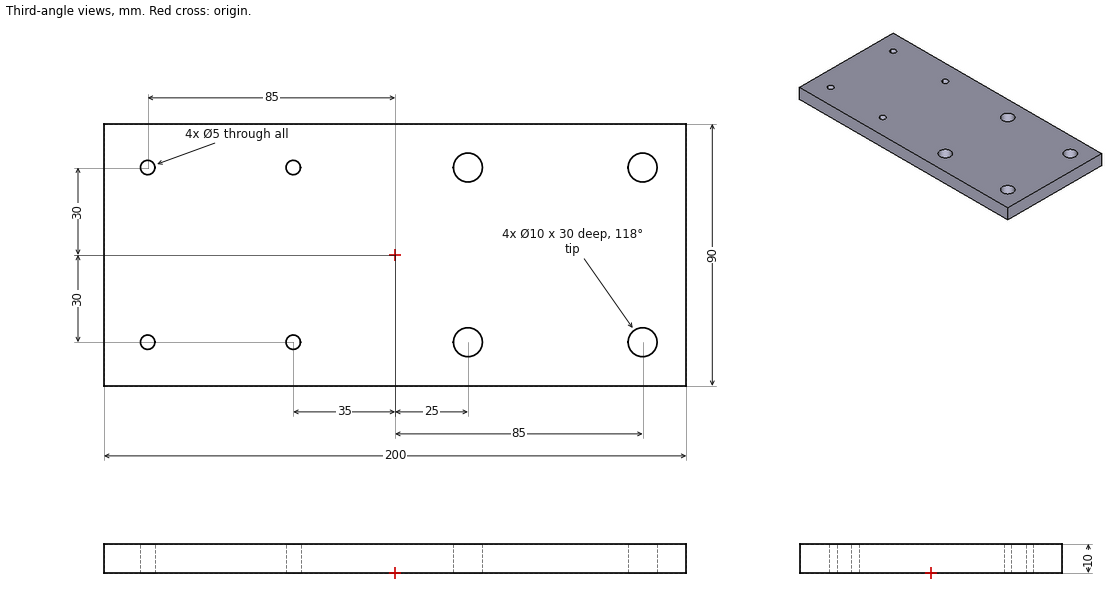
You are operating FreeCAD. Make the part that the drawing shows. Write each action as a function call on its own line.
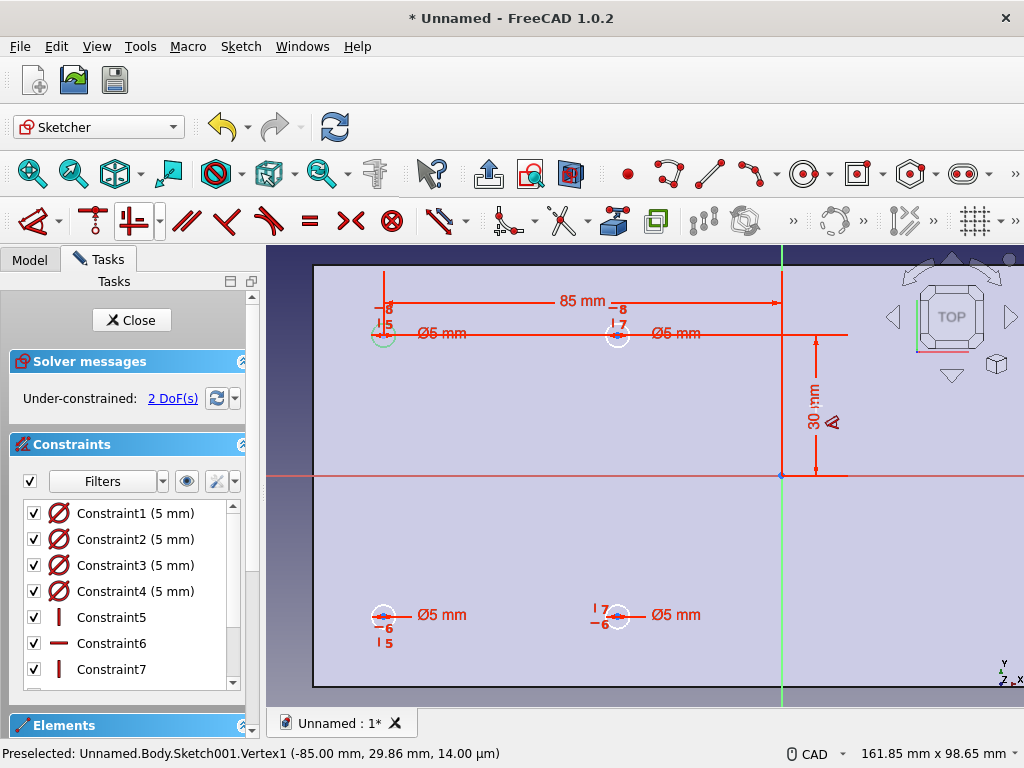
click(618, 617)
click(700, 651)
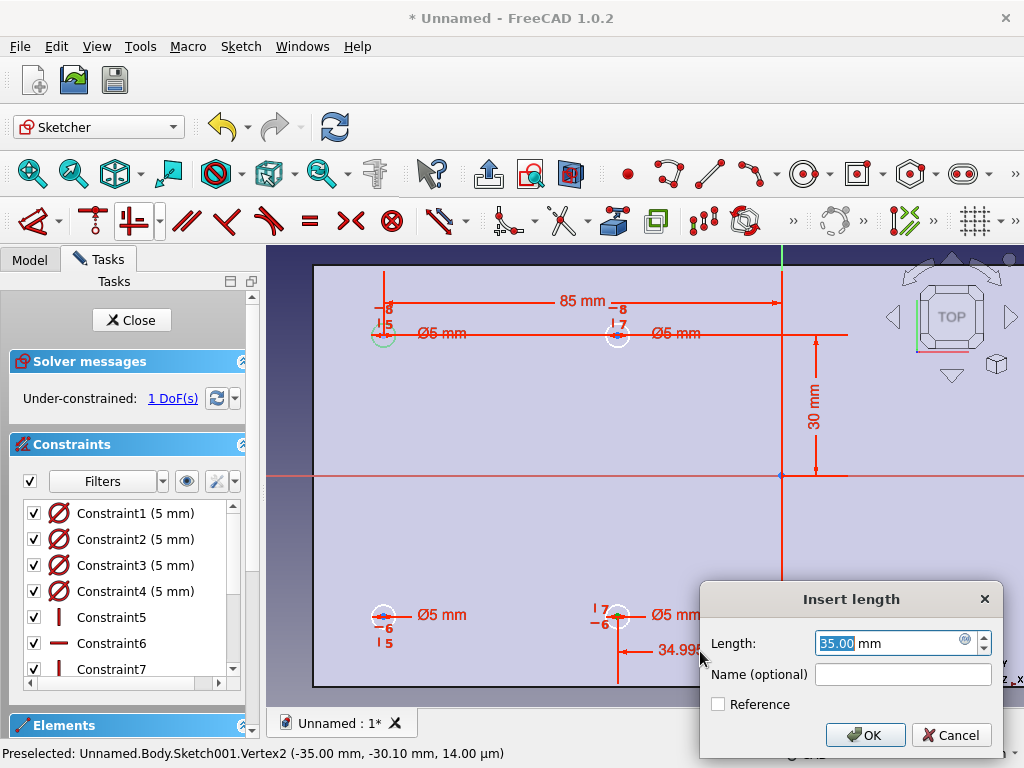
text(35)
key(Return)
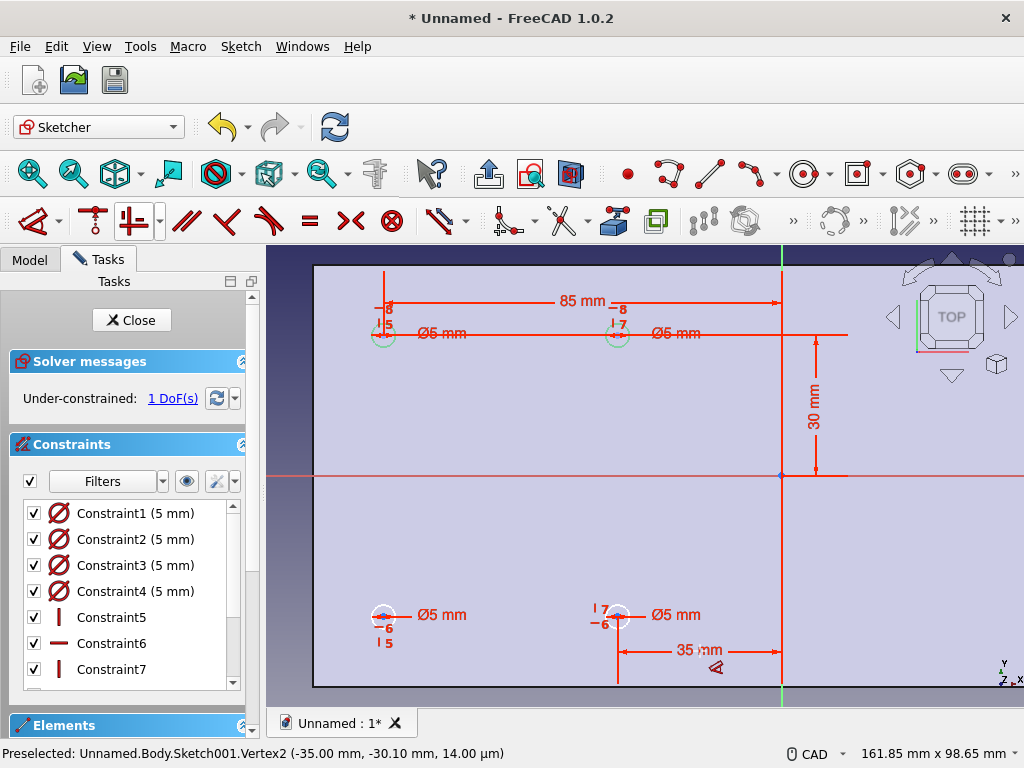
click(618, 617)
click(816, 546)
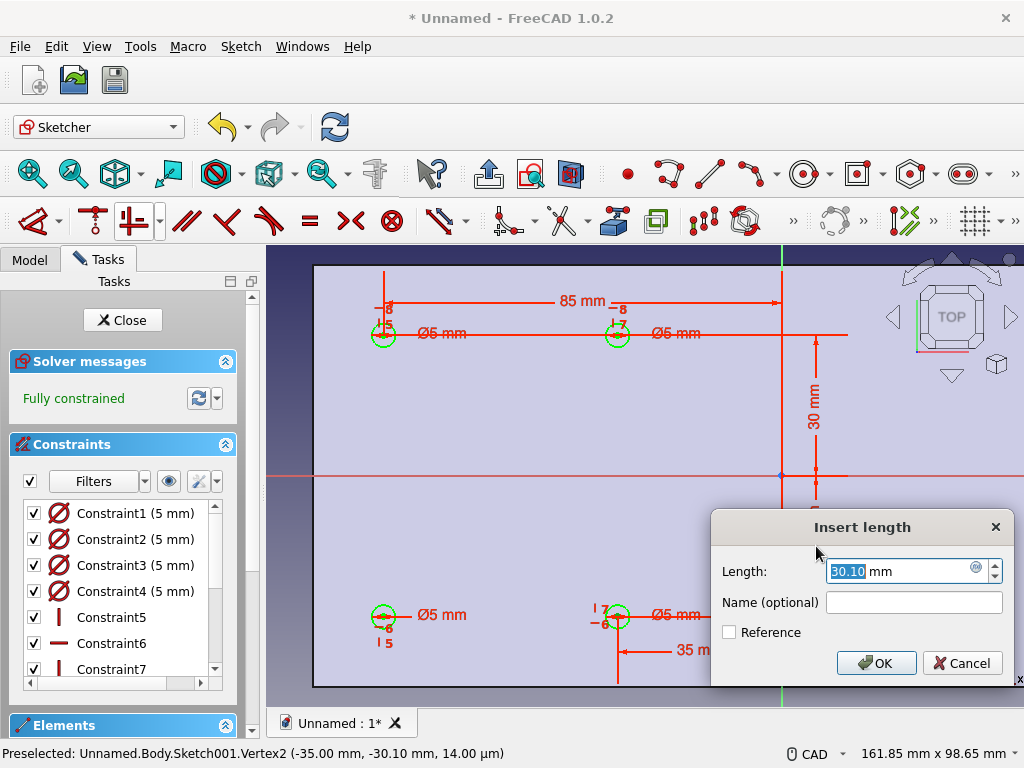
text(30)
key(Return)
key(Escape)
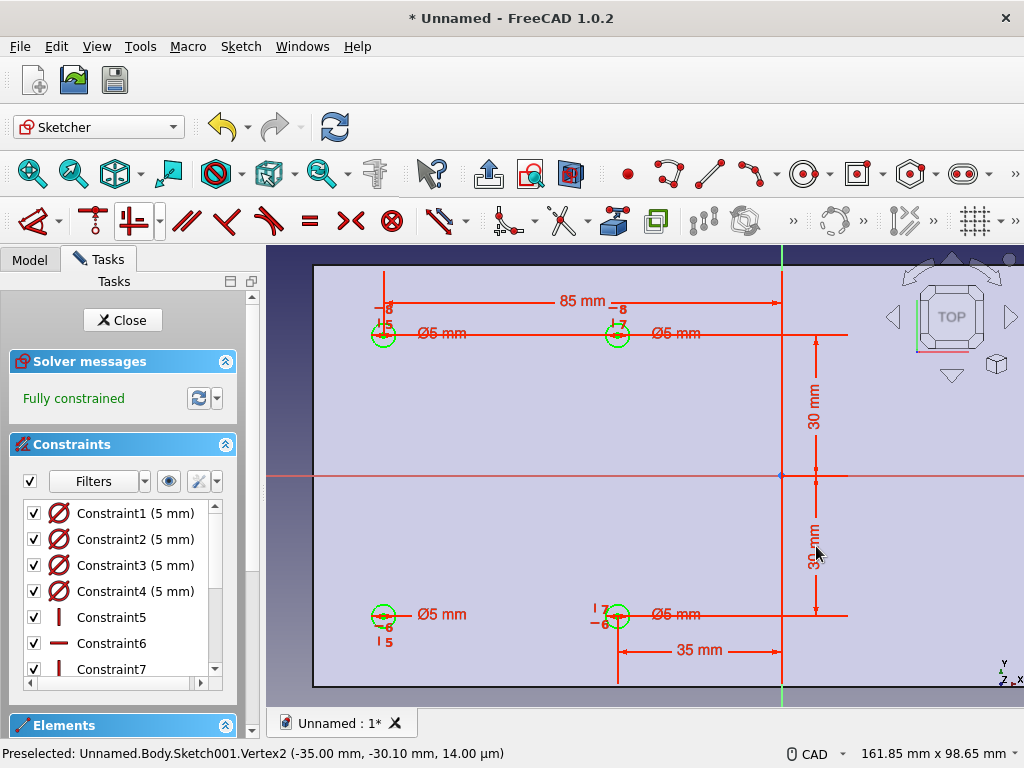
click(123, 320)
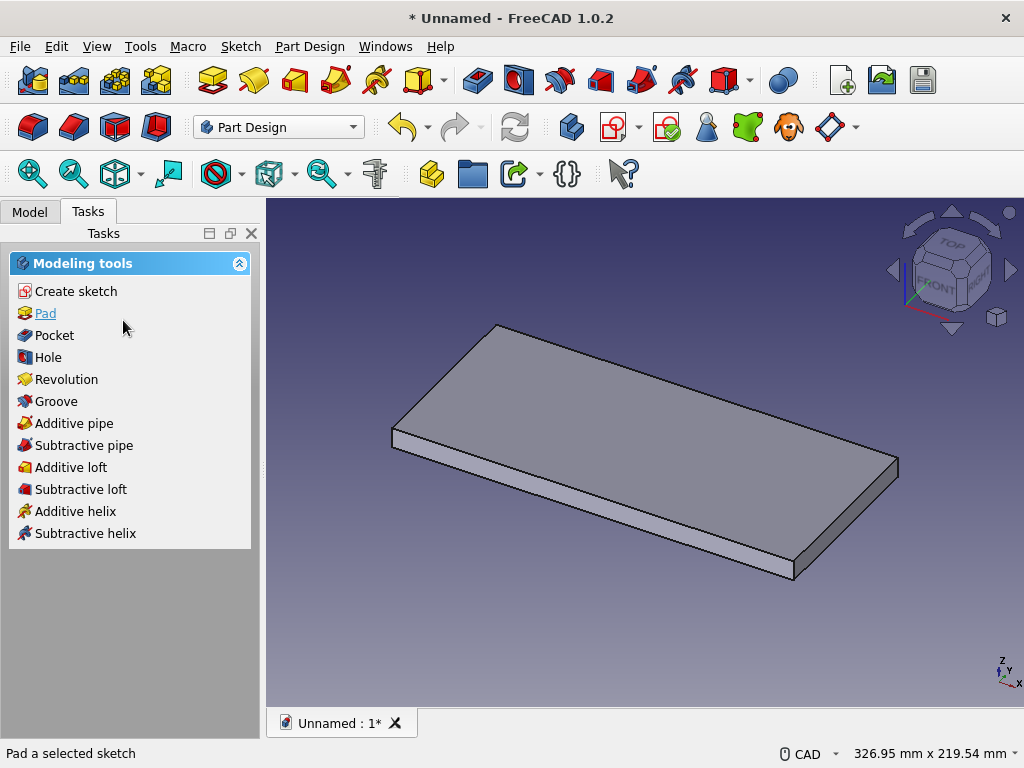
click(519, 80)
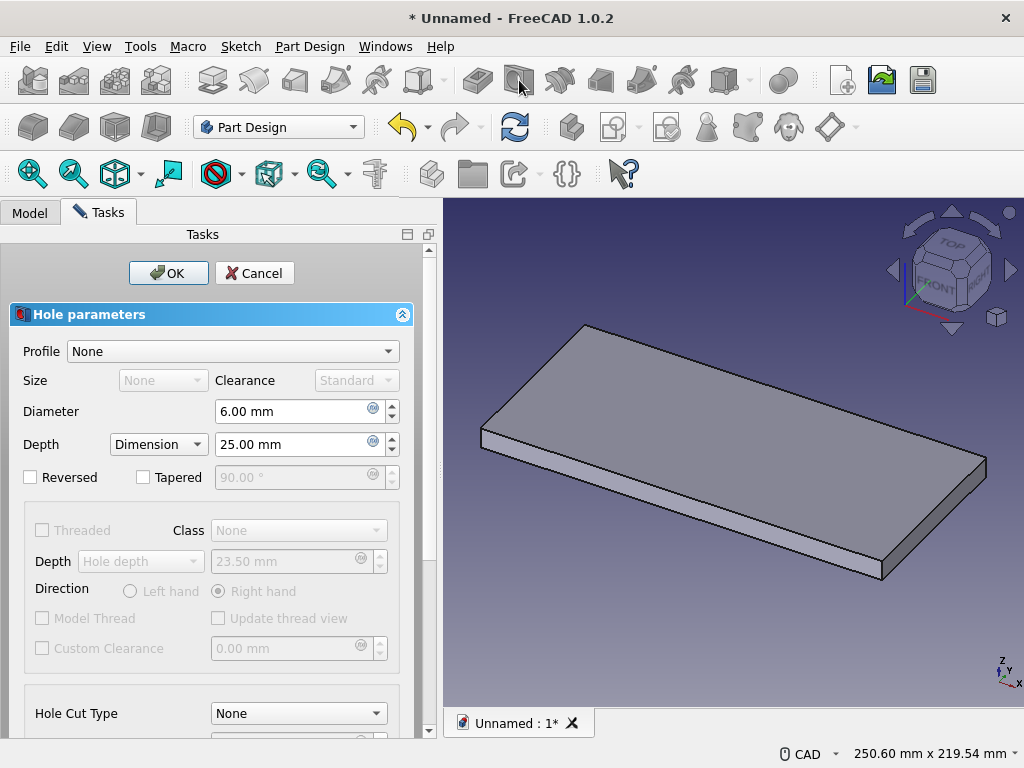
triple_click(300, 412)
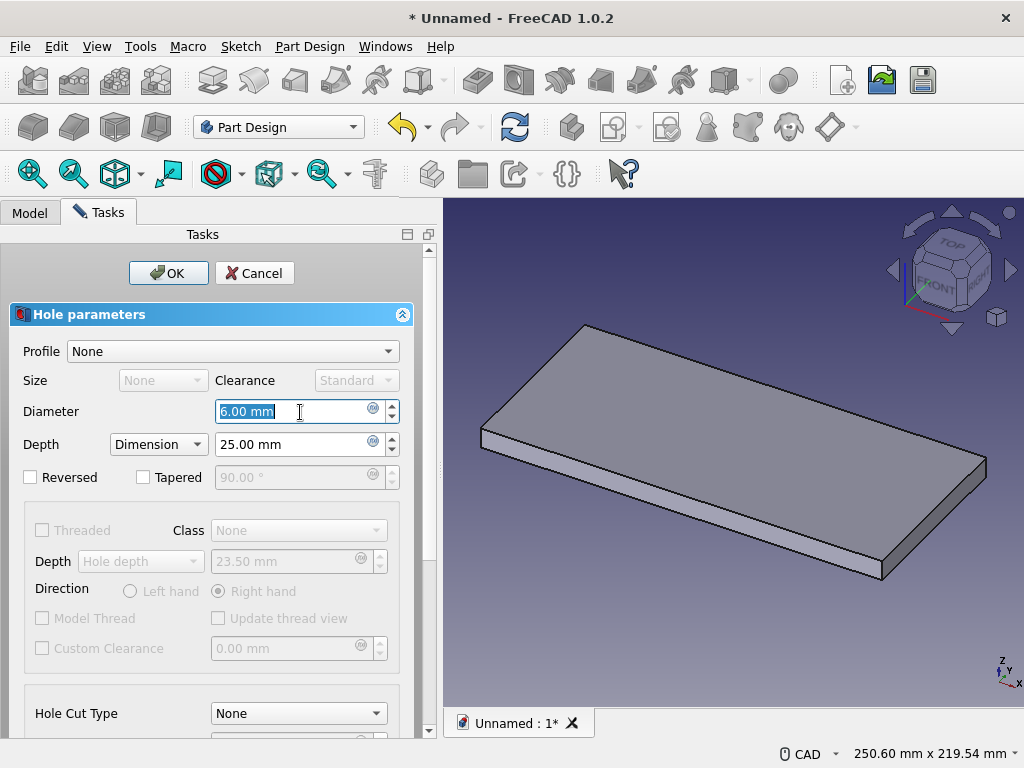
text(5)
key(Tab)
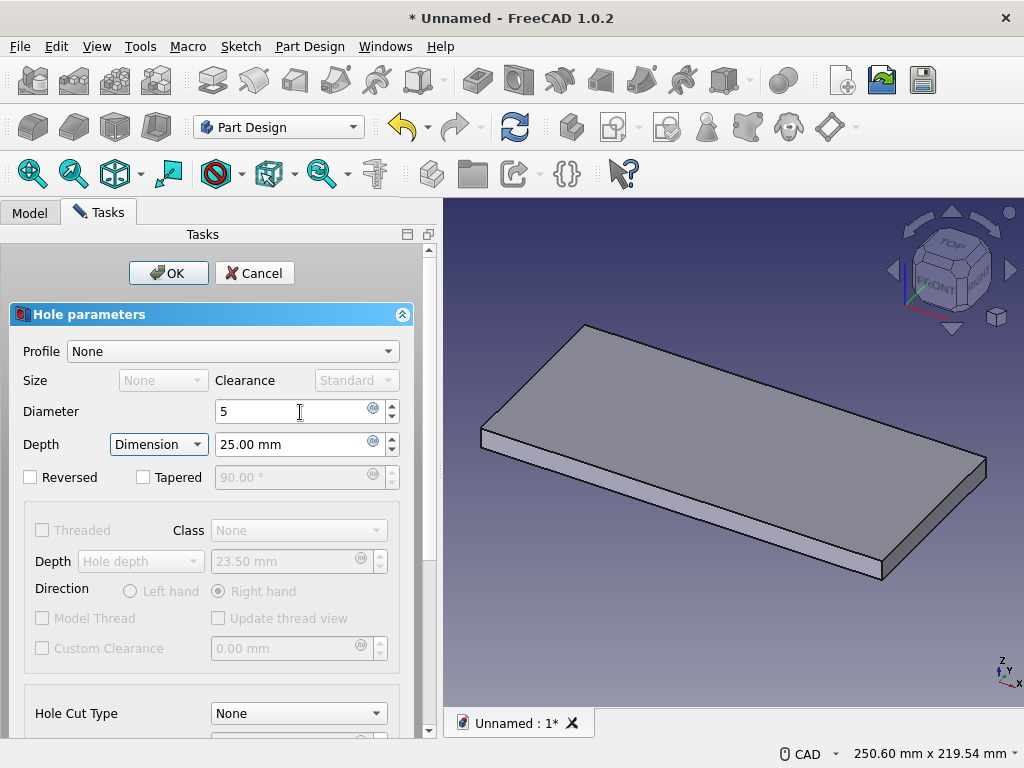
click(160, 444)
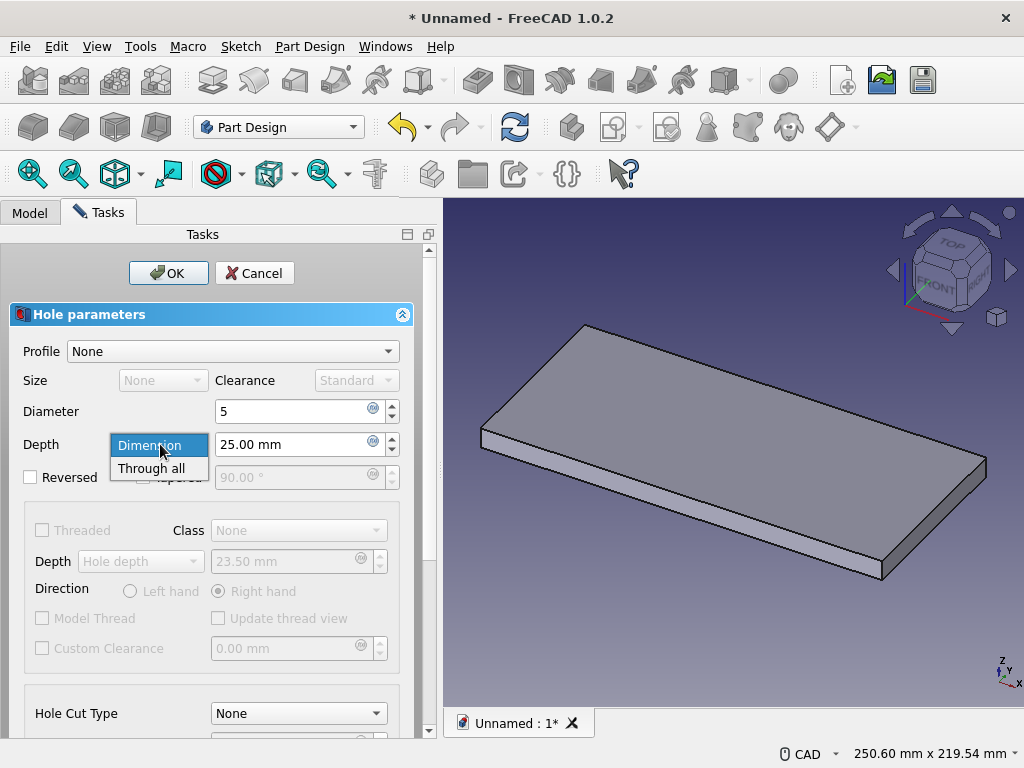
click(158, 468)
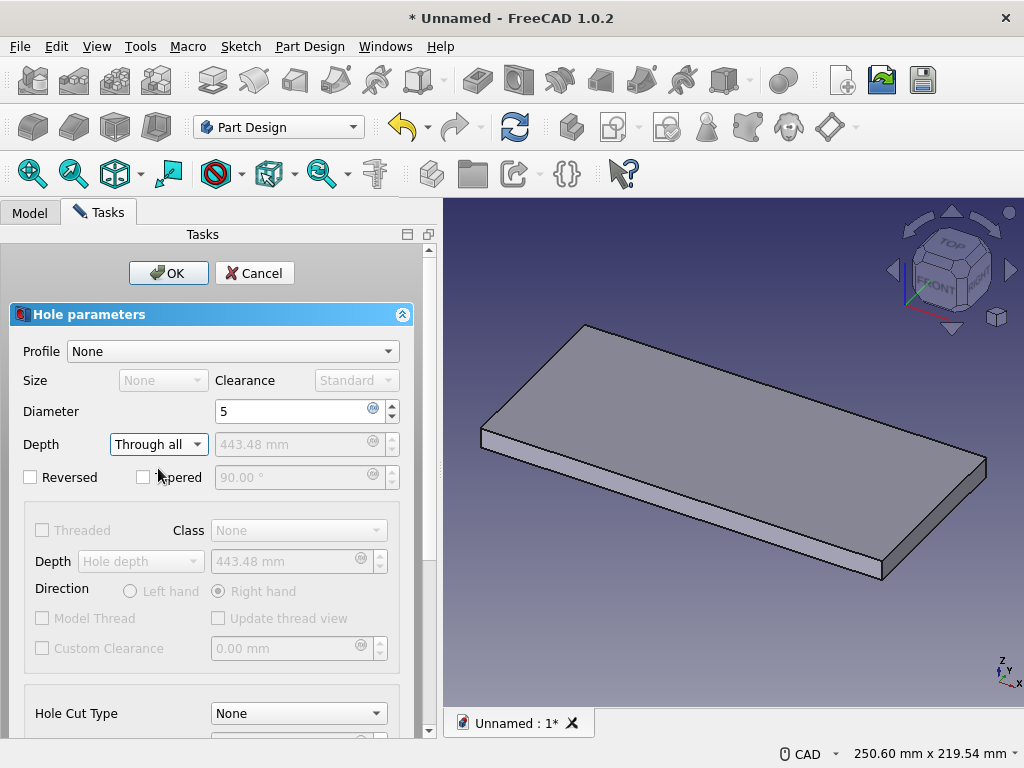
click(31, 477)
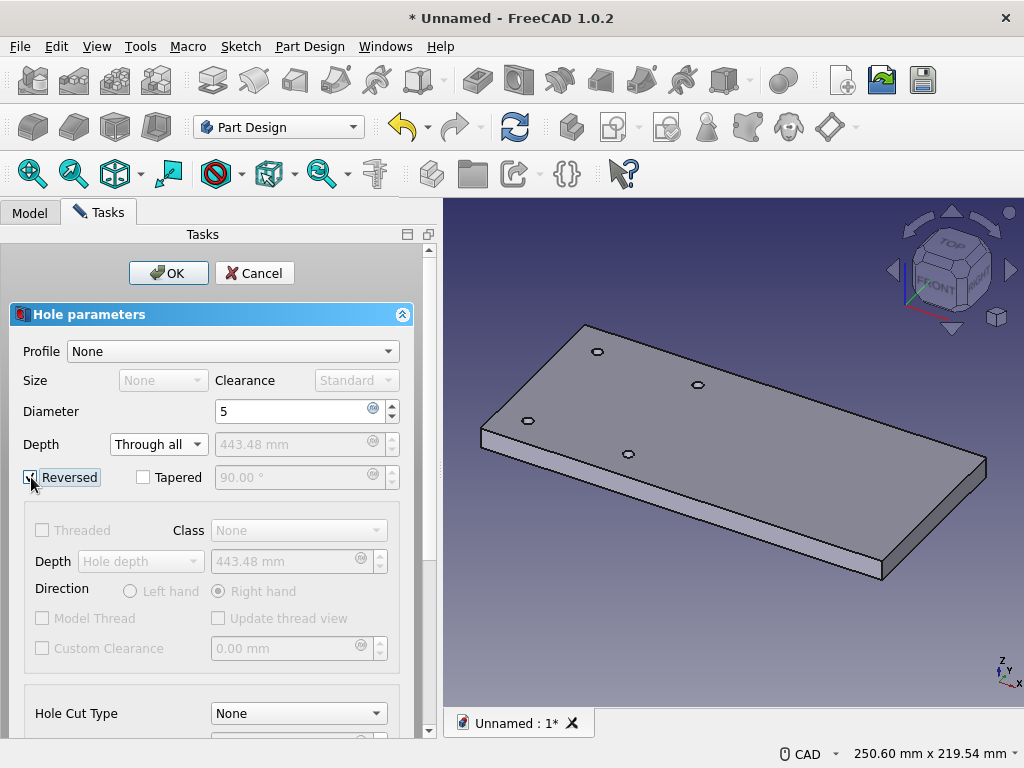
click(169, 273)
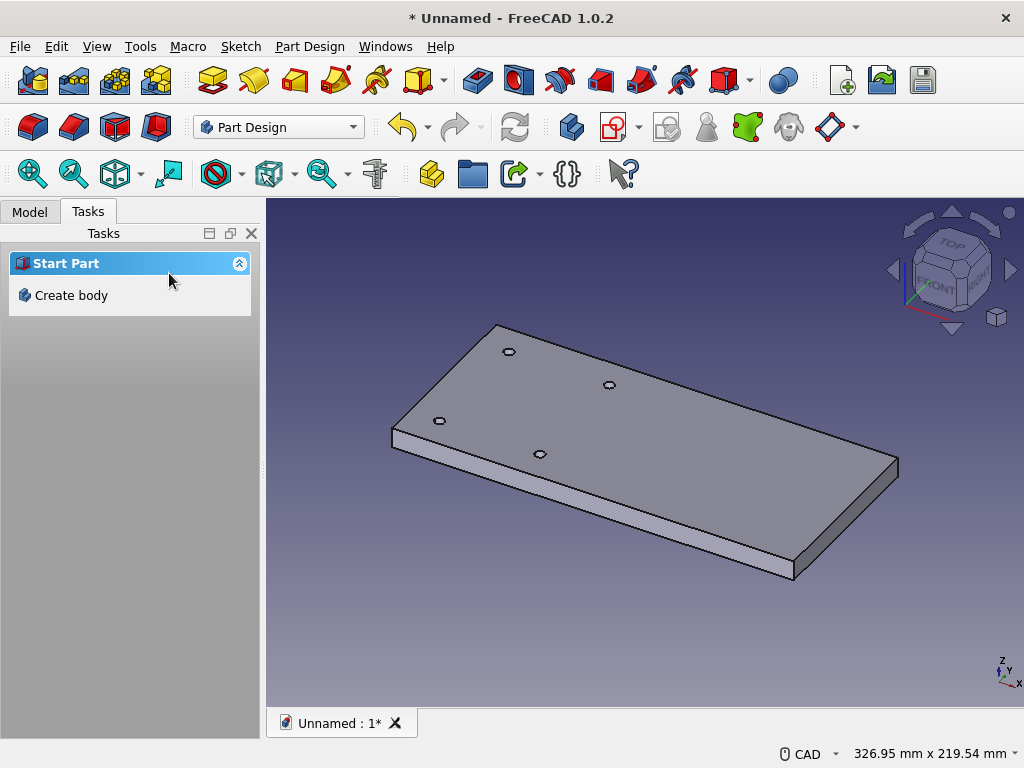
click(702, 461)